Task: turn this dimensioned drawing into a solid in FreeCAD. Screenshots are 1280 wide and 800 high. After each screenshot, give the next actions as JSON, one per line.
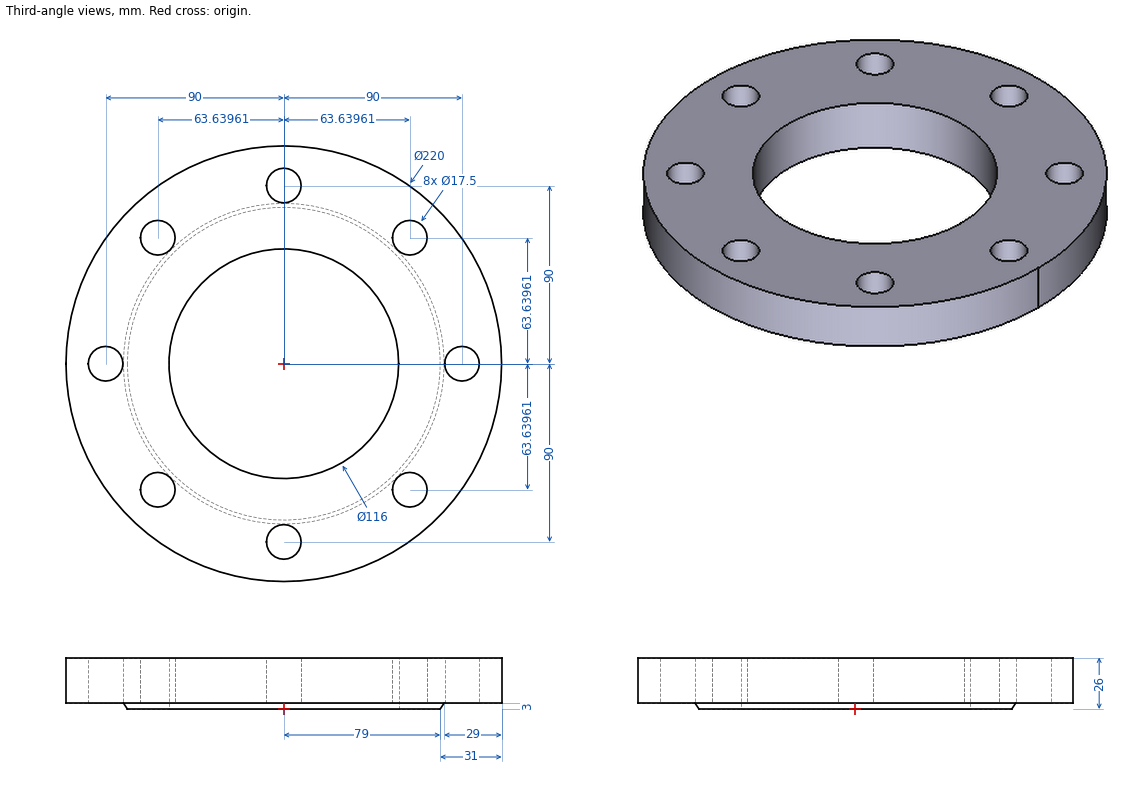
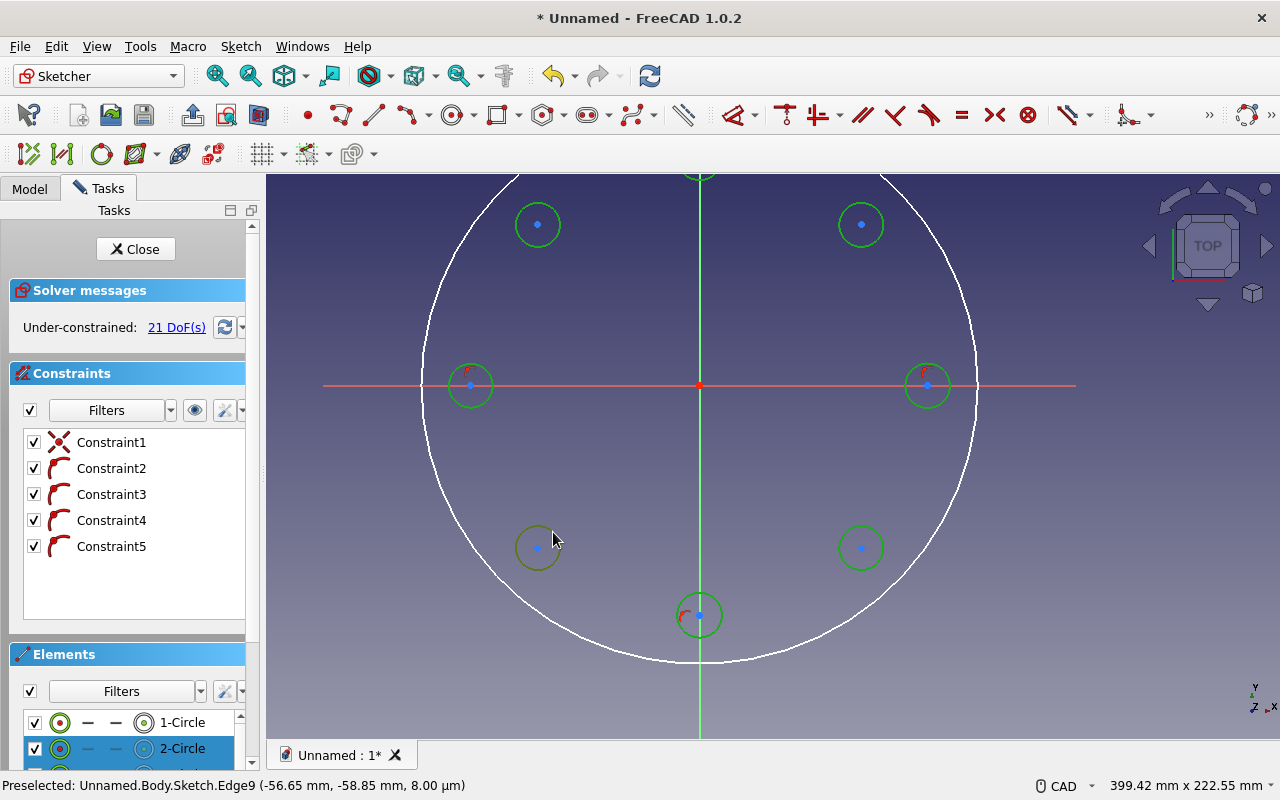
{"action": "left_click", "coordinate": [962, 116]}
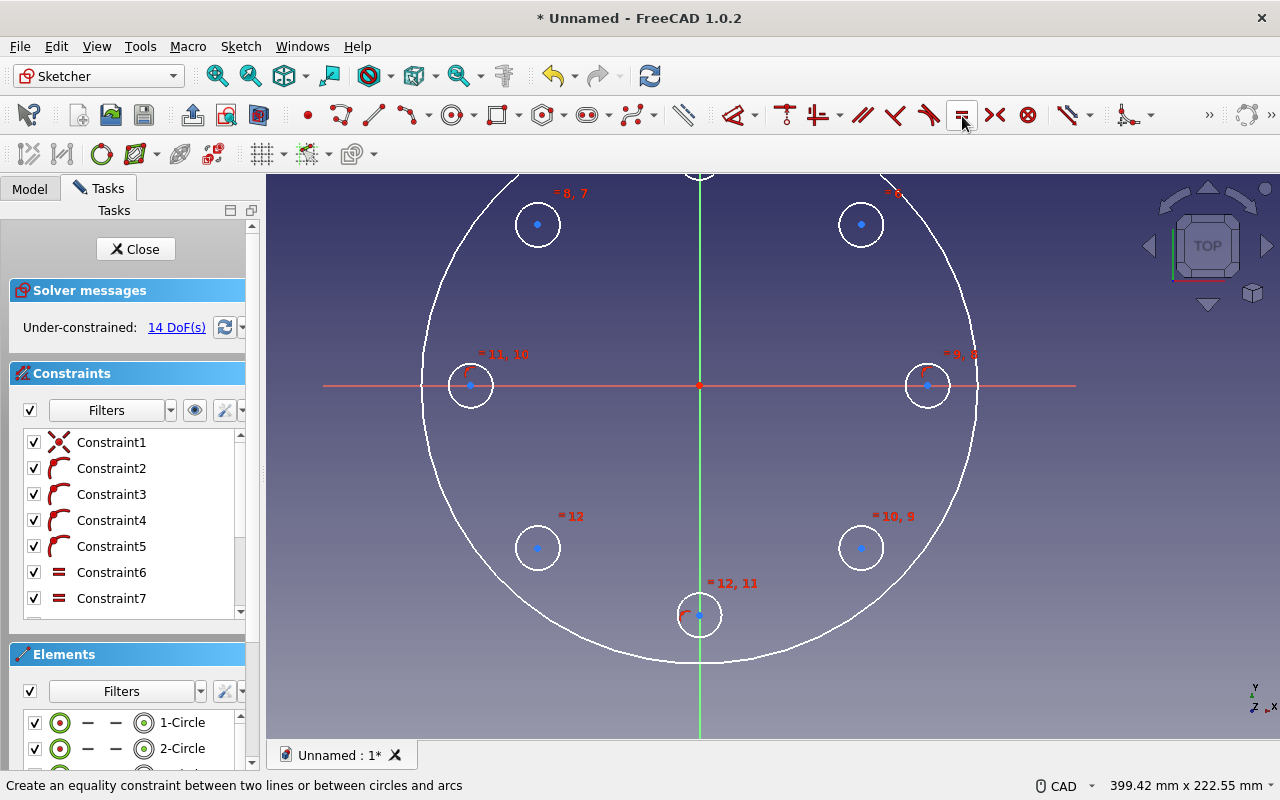
{"action": "left_click", "coordinate": [861, 225]}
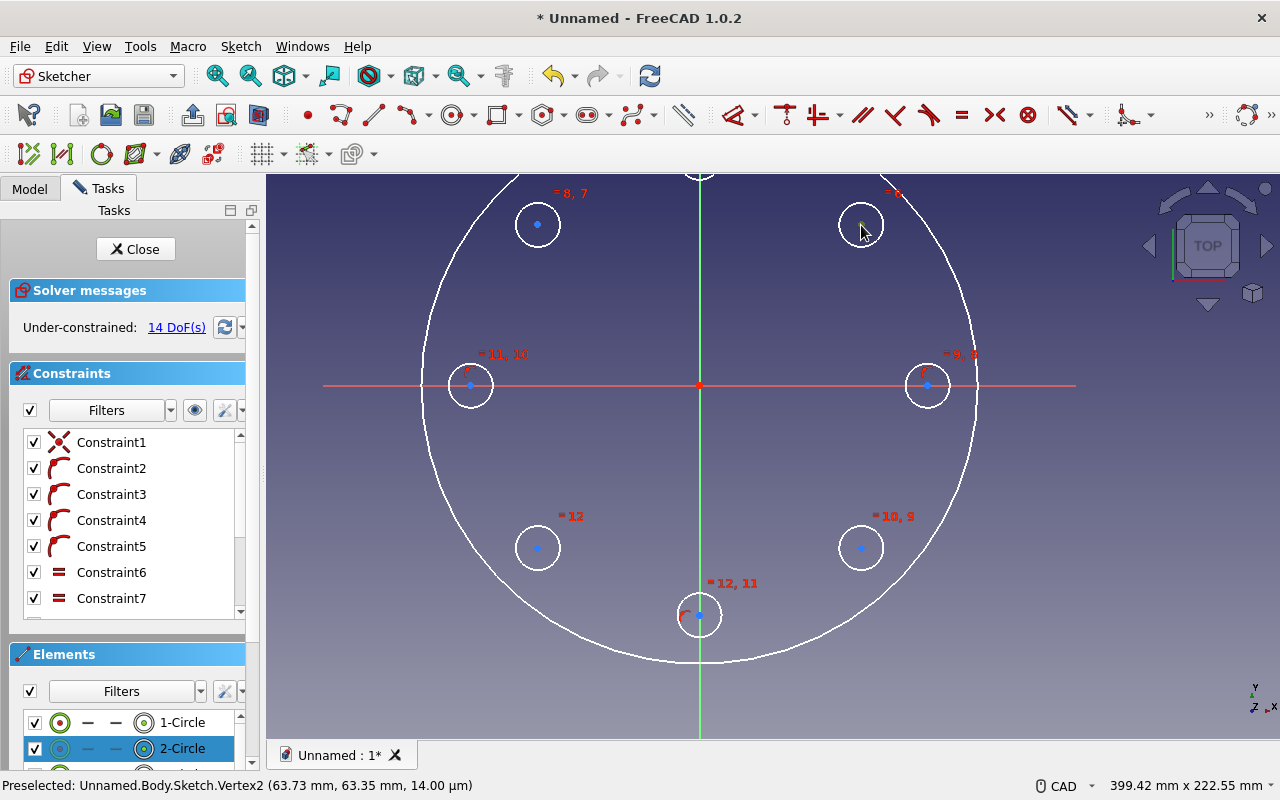
{"action": "left_click", "coordinate": [538, 225]}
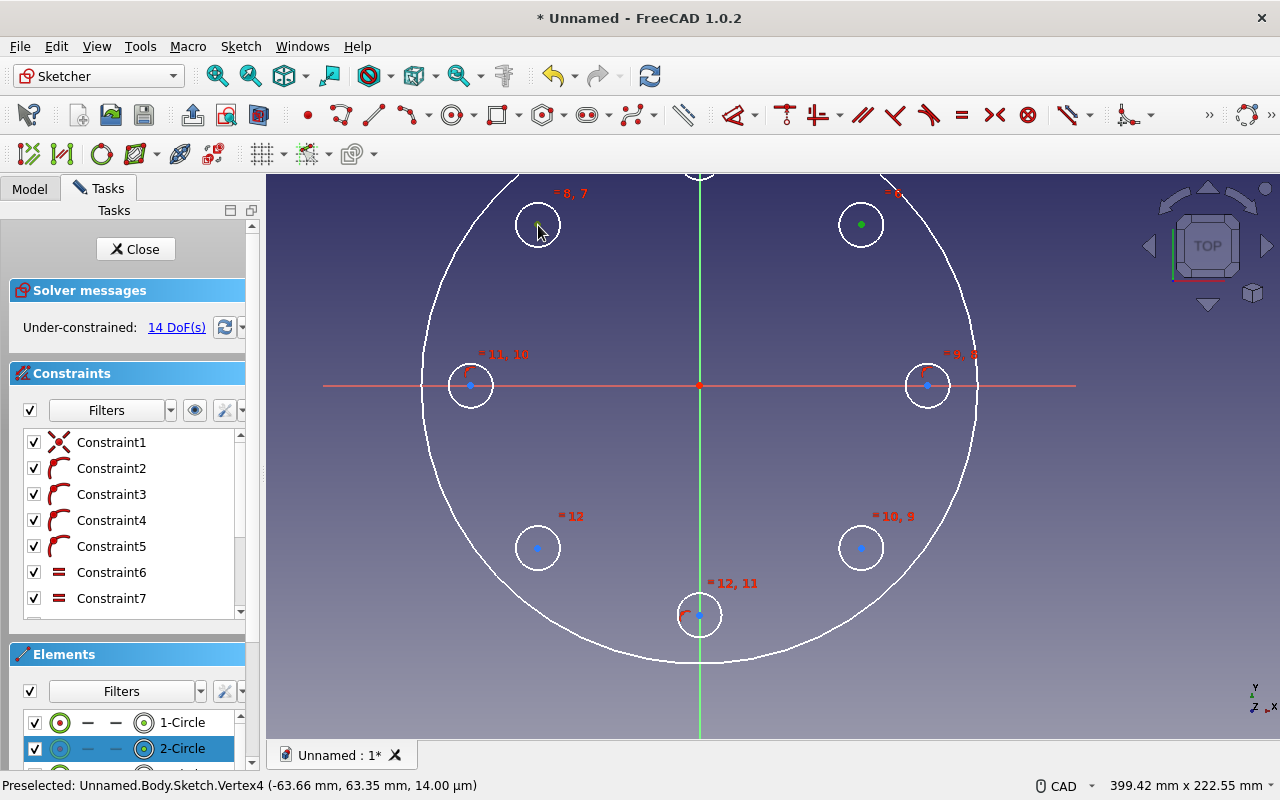
{"action": "left_click", "coordinate": [840, 116]}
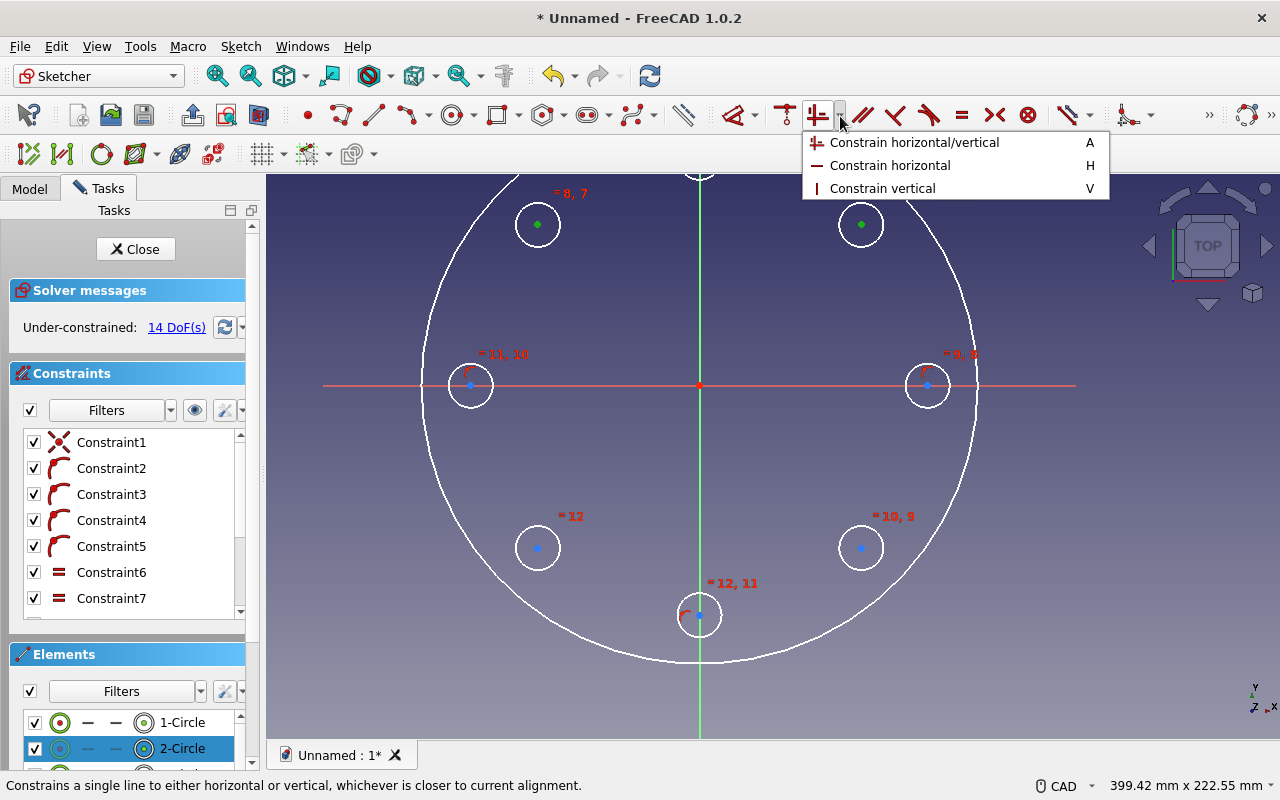
{"action": "left_click", "coordinate": [956, 166]}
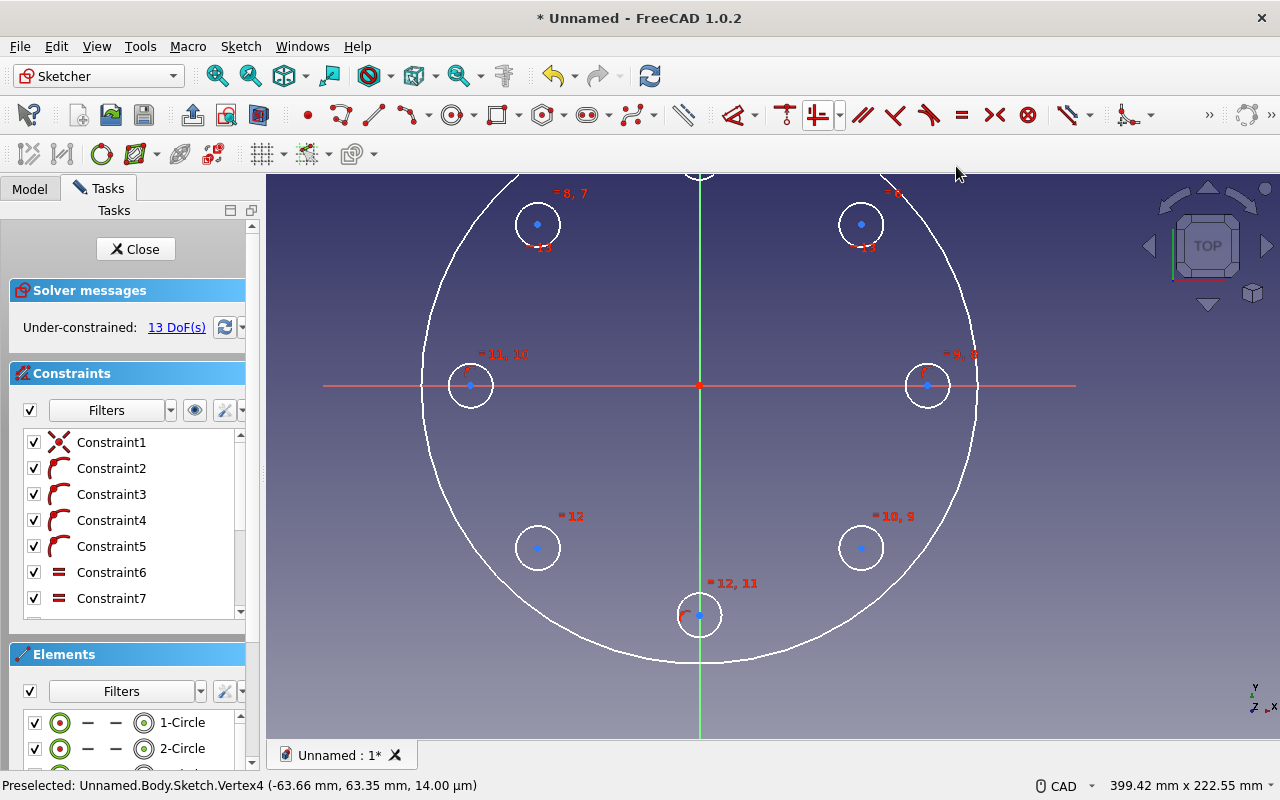
{"action": "left_click", "coordinate": [861, 225]}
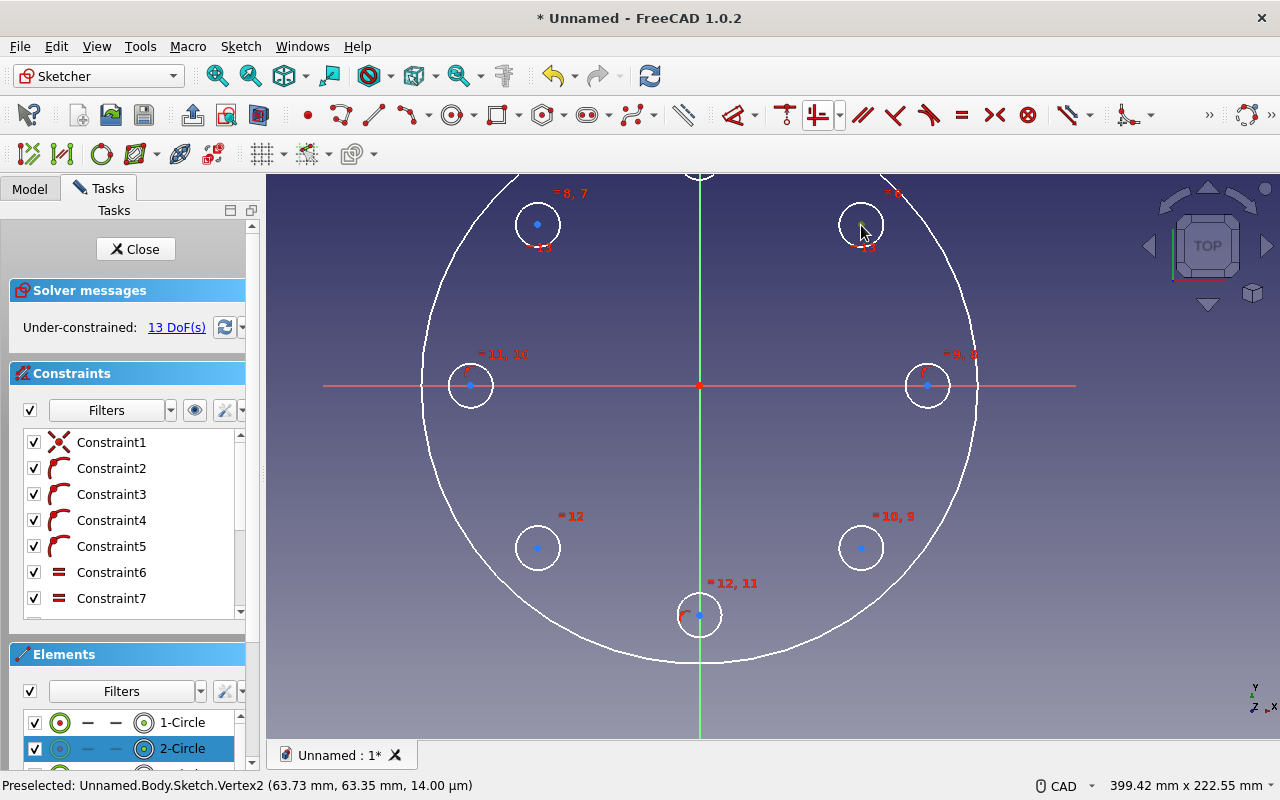
{"action": "left_click", "coordinate": [861, 548]}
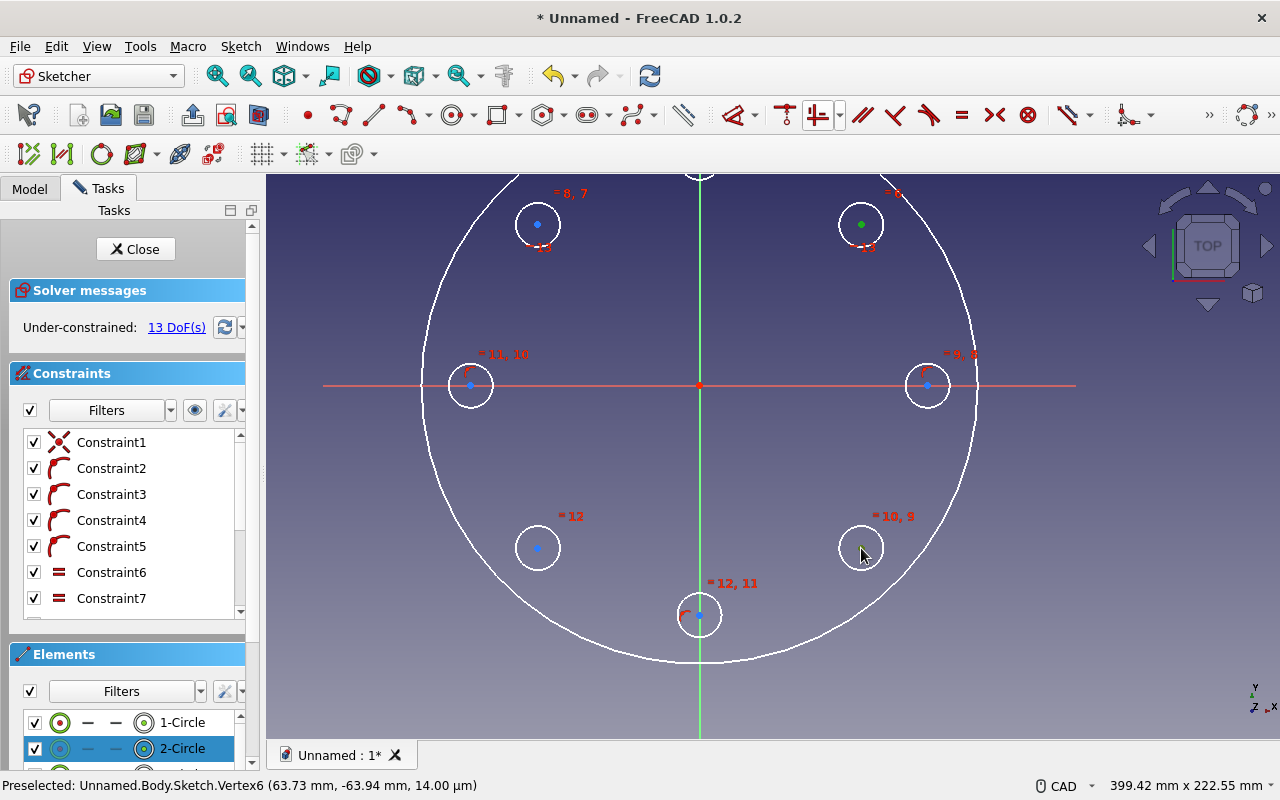
{"action": "key", "text": "v"}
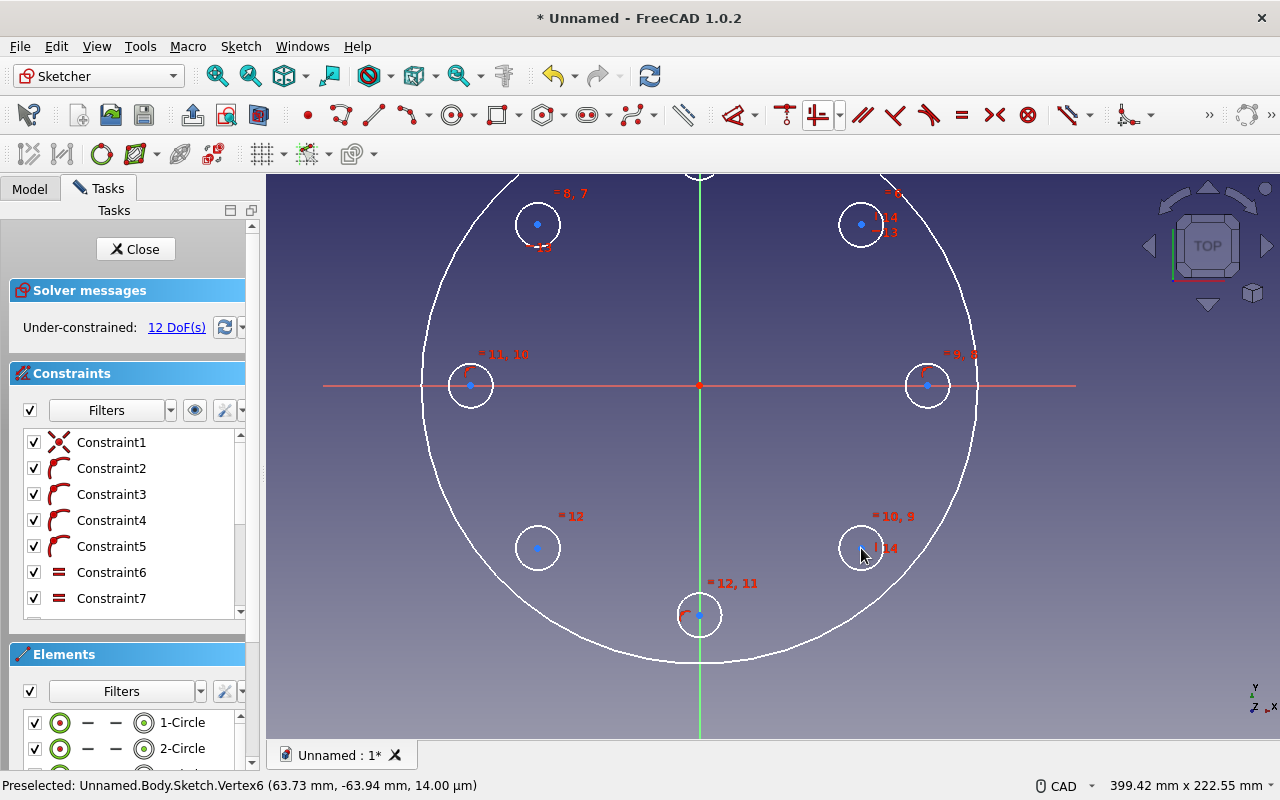
{"action": "left_click", "coordinate": [538, 225]}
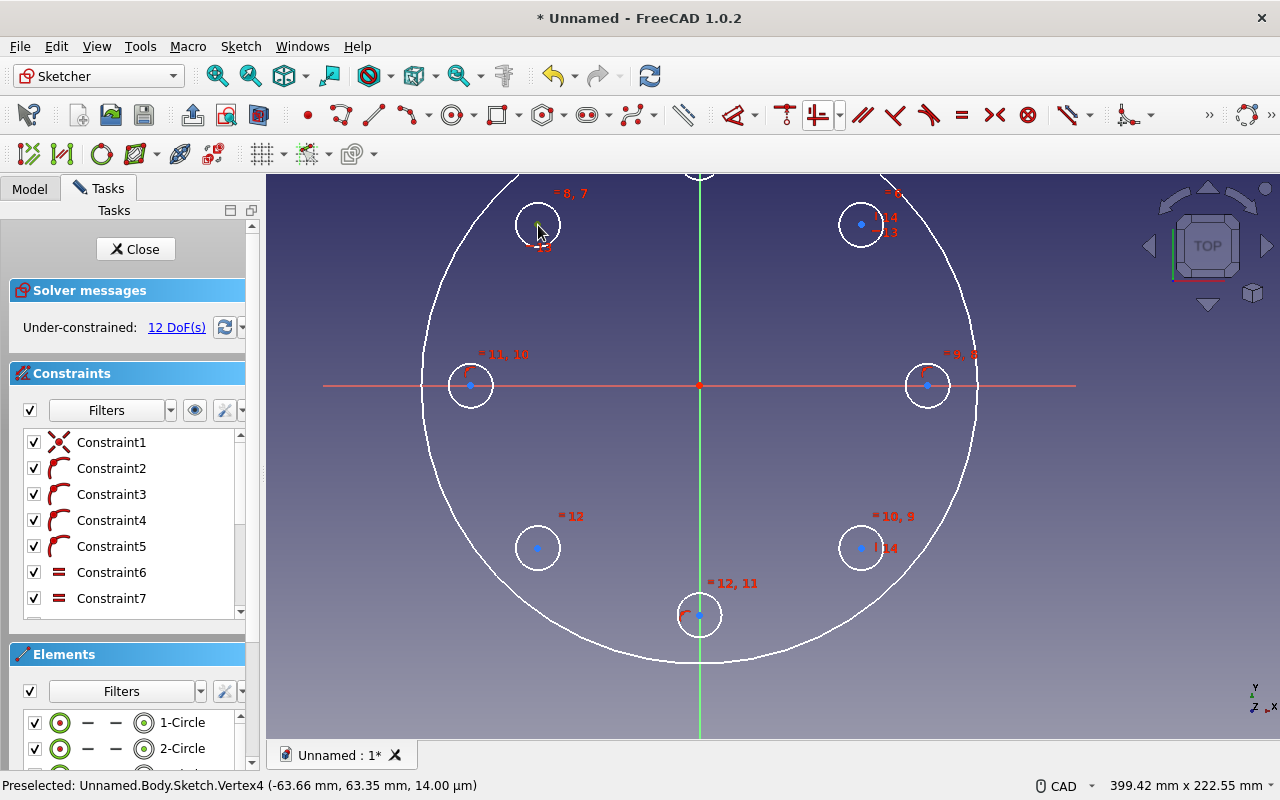
{"action": "left_click", "coordinate": [538, 548]}